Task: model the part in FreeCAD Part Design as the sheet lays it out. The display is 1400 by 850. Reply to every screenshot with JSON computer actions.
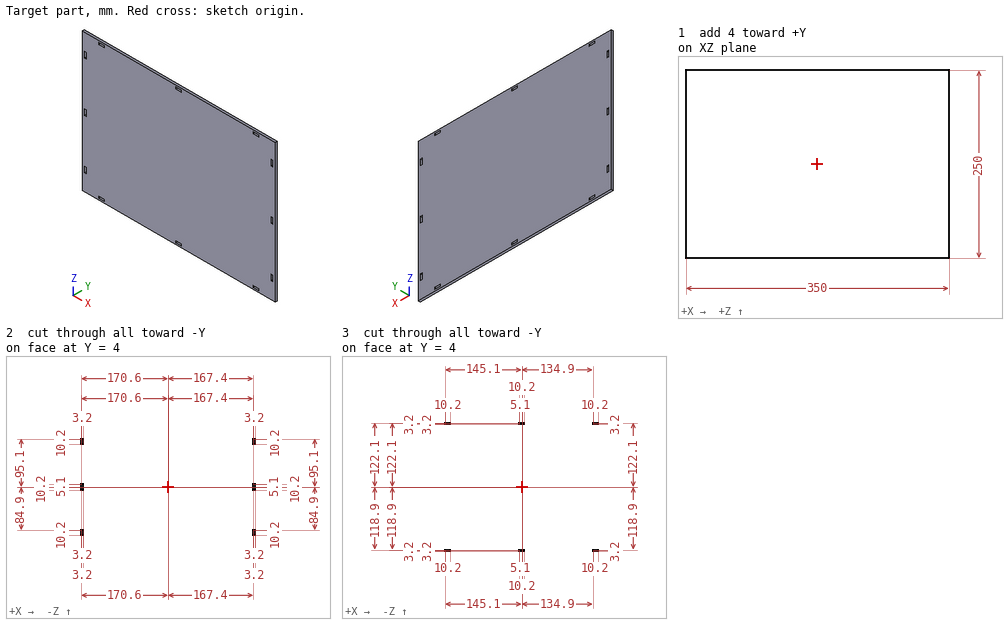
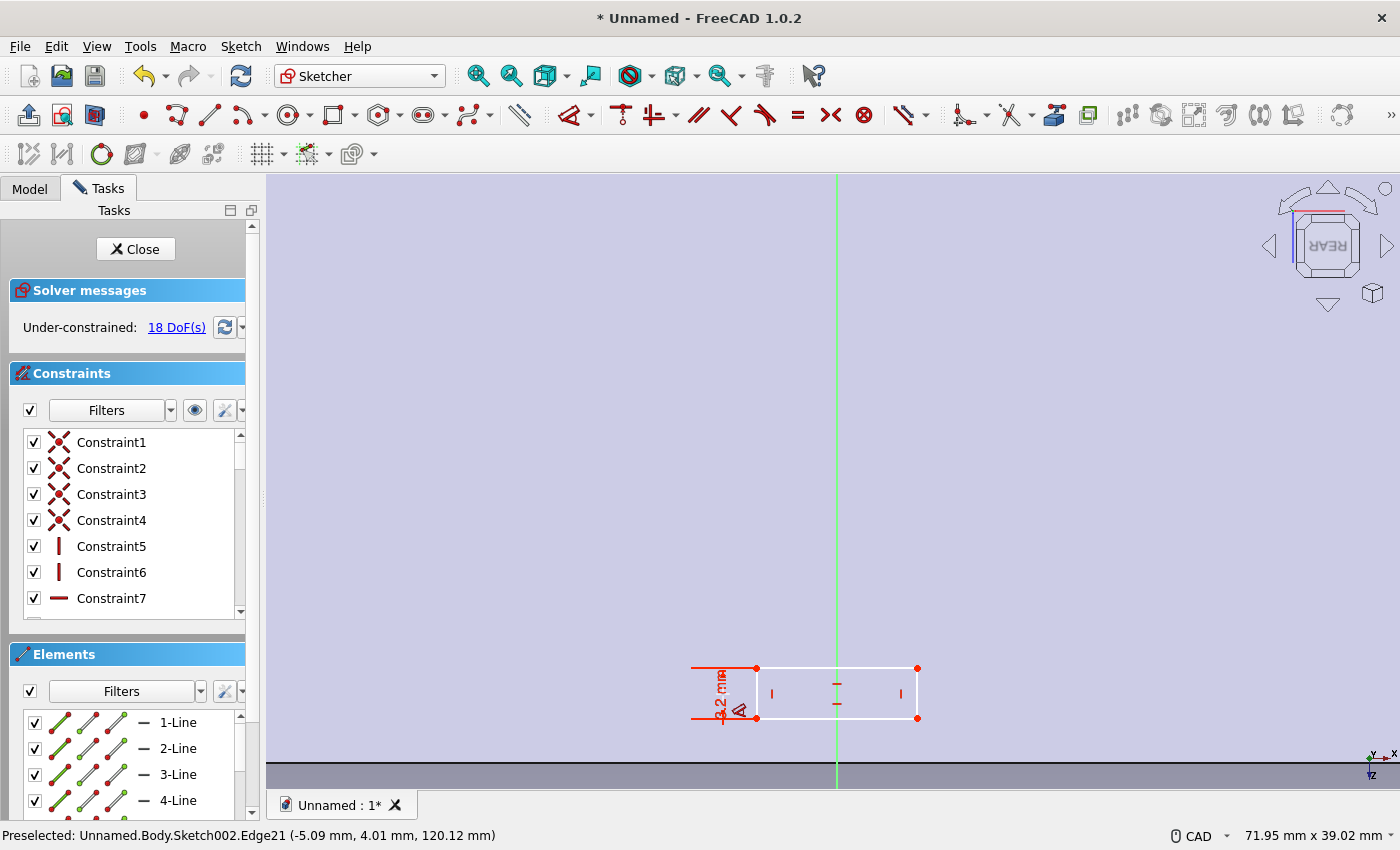
{"action": "scroll", "coordinate": [755, 692], "scroll_direction": "down", "scroll_amount": 11}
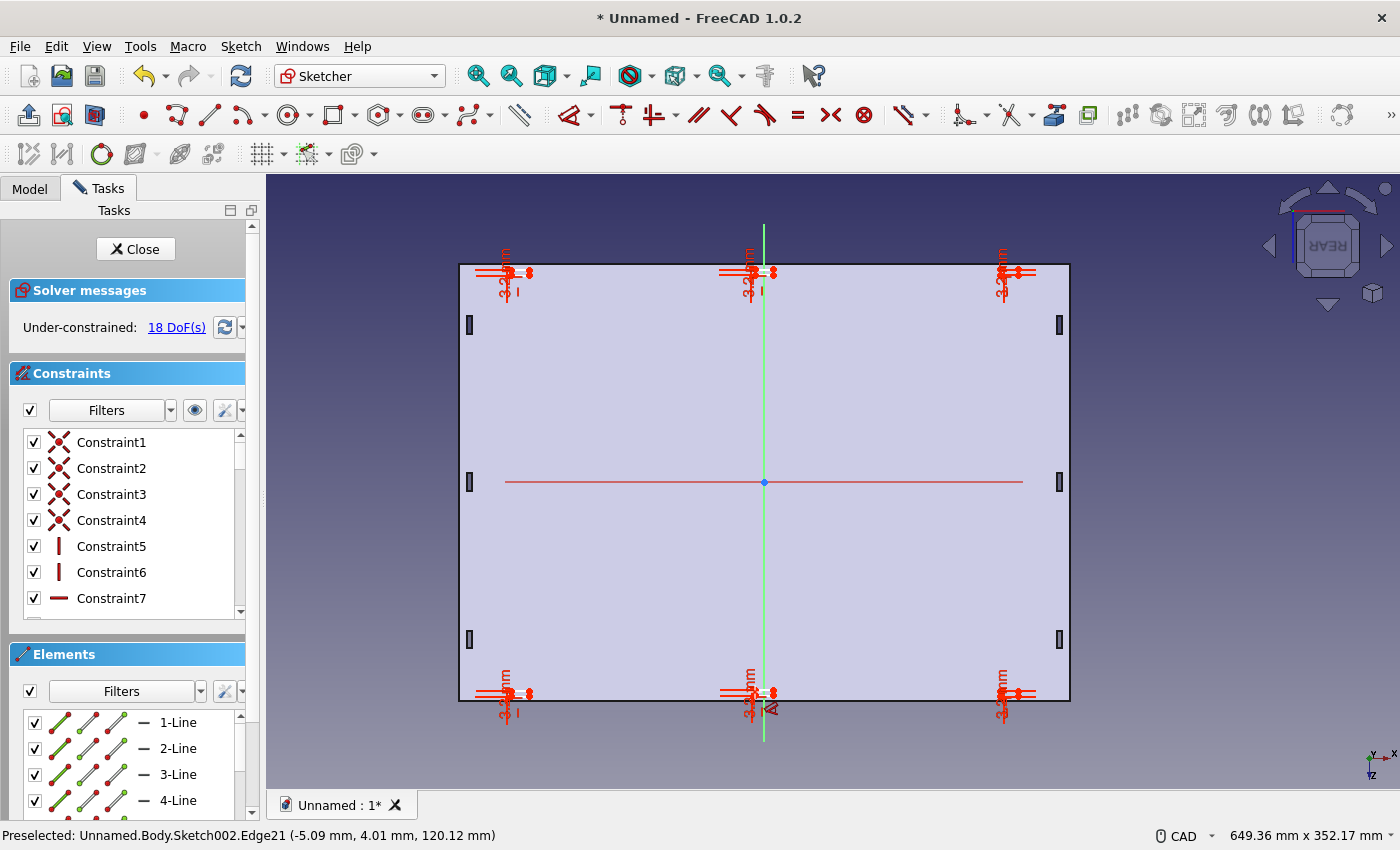
{"action": "scroll", "coordinate": [761, 275], "scroll_direction": "up", "scroll_amount": 7}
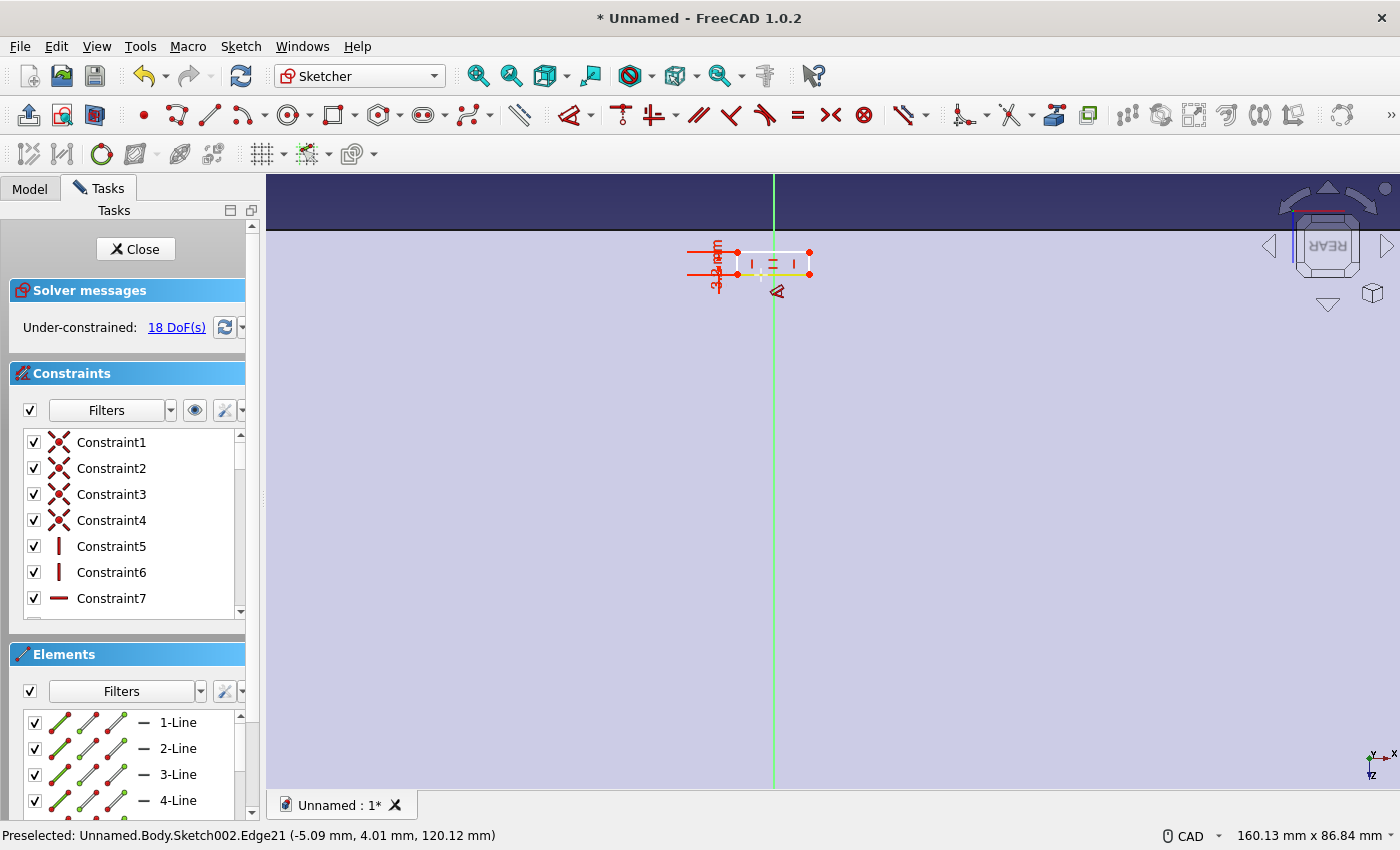
{"action": "left_click", "coordinate": [759, 275]}
{"action": "left_click", "coordinate": [757, 309]}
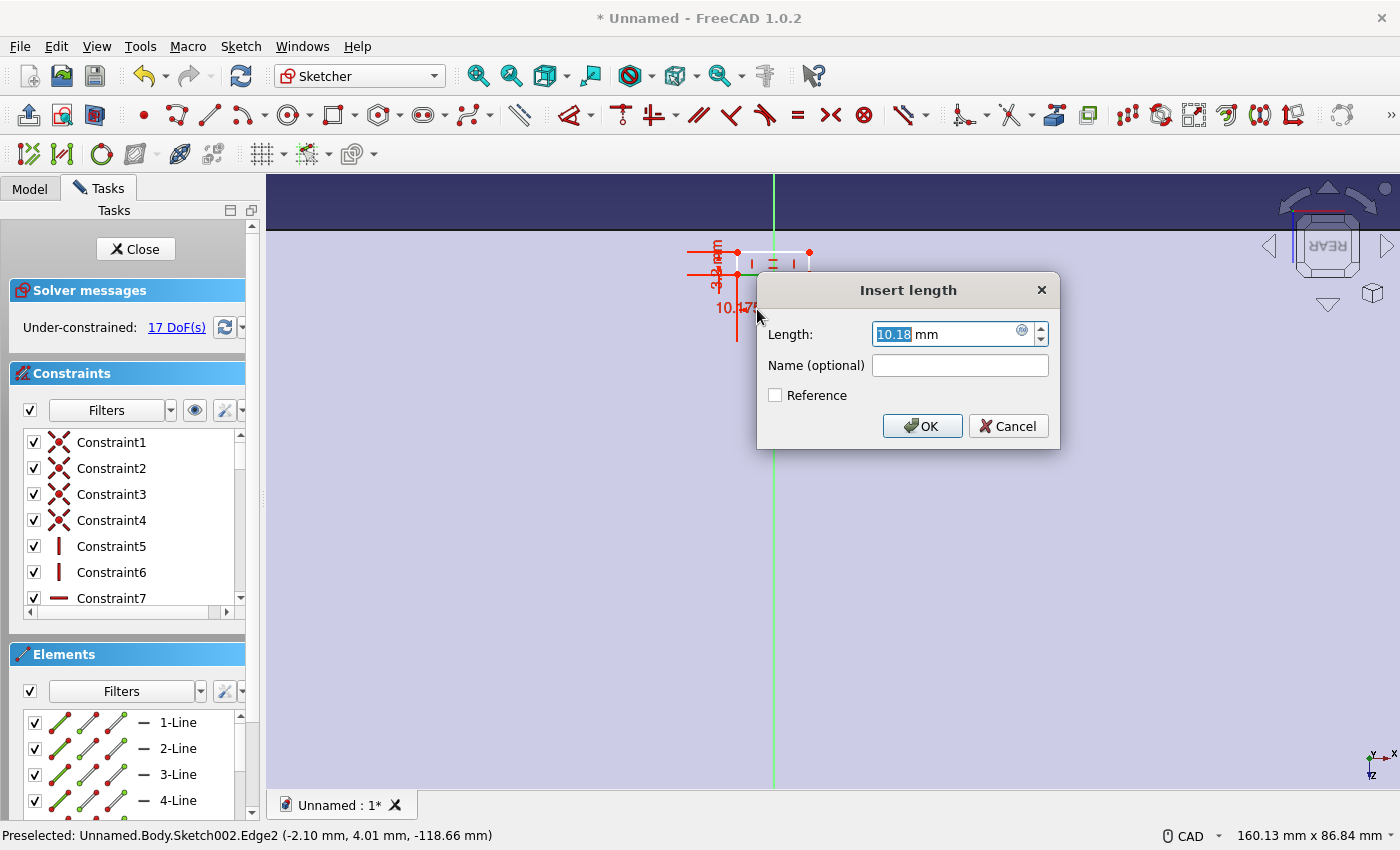
{"action": "type", "text": "10.2"}
{"action": "key", "text": "Return"}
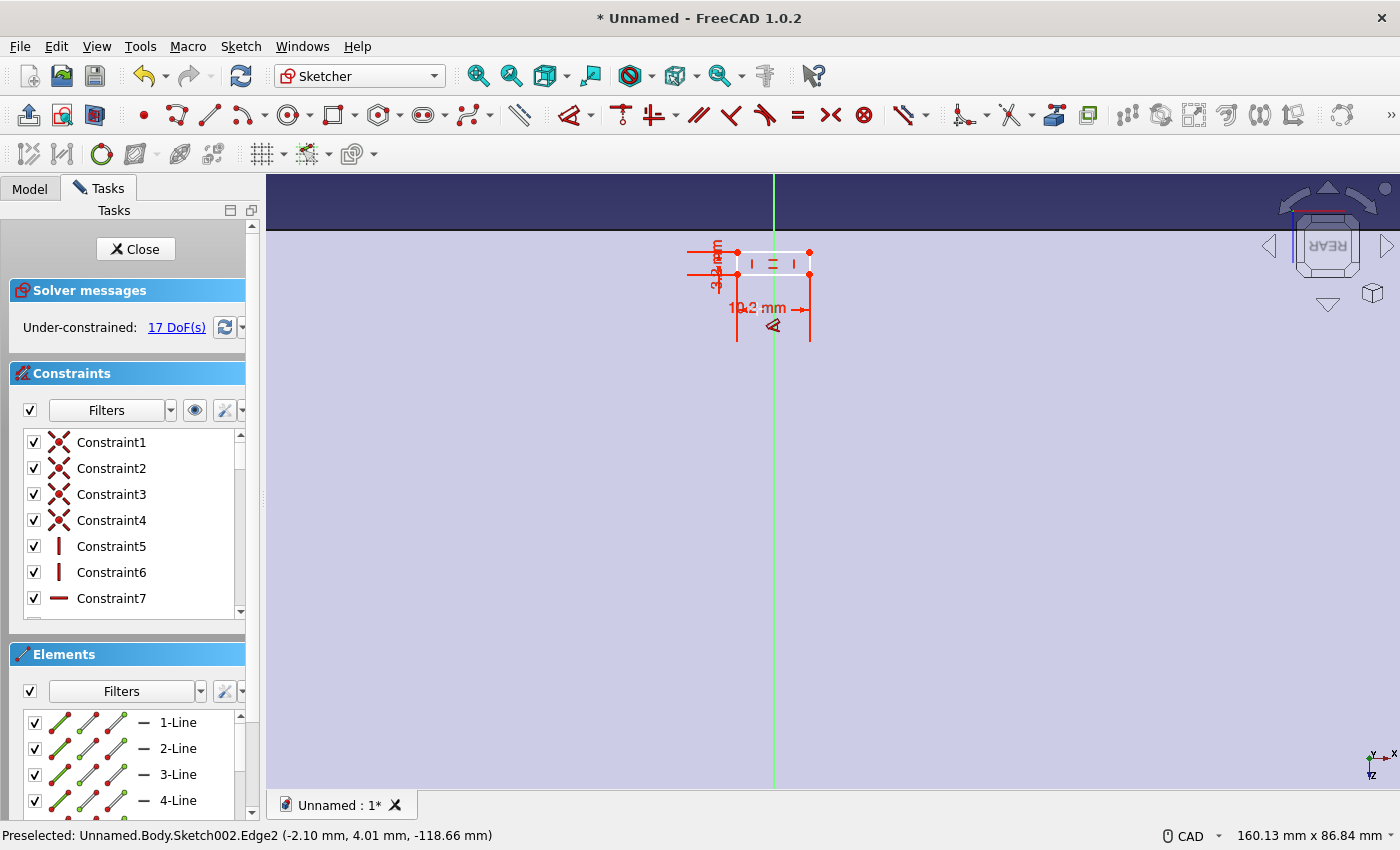
{"action": "scroll", "coordinate": [761, 274], "scroll_direction": "down", "scroll_amount": 7}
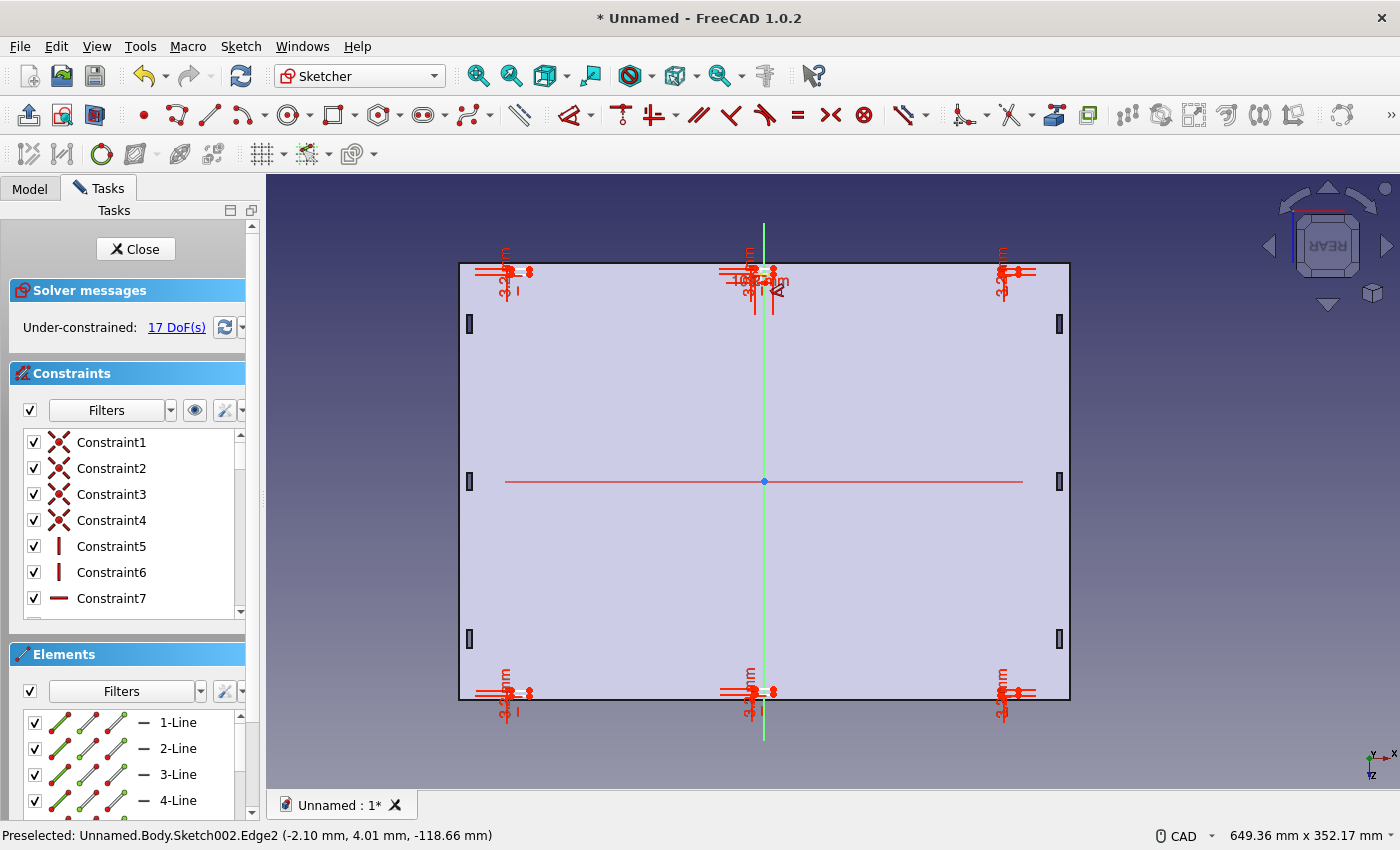
{"action": "scroll", "coordinate": [1006, 275], "scroll_direction": "up", "scroll_amount": 5}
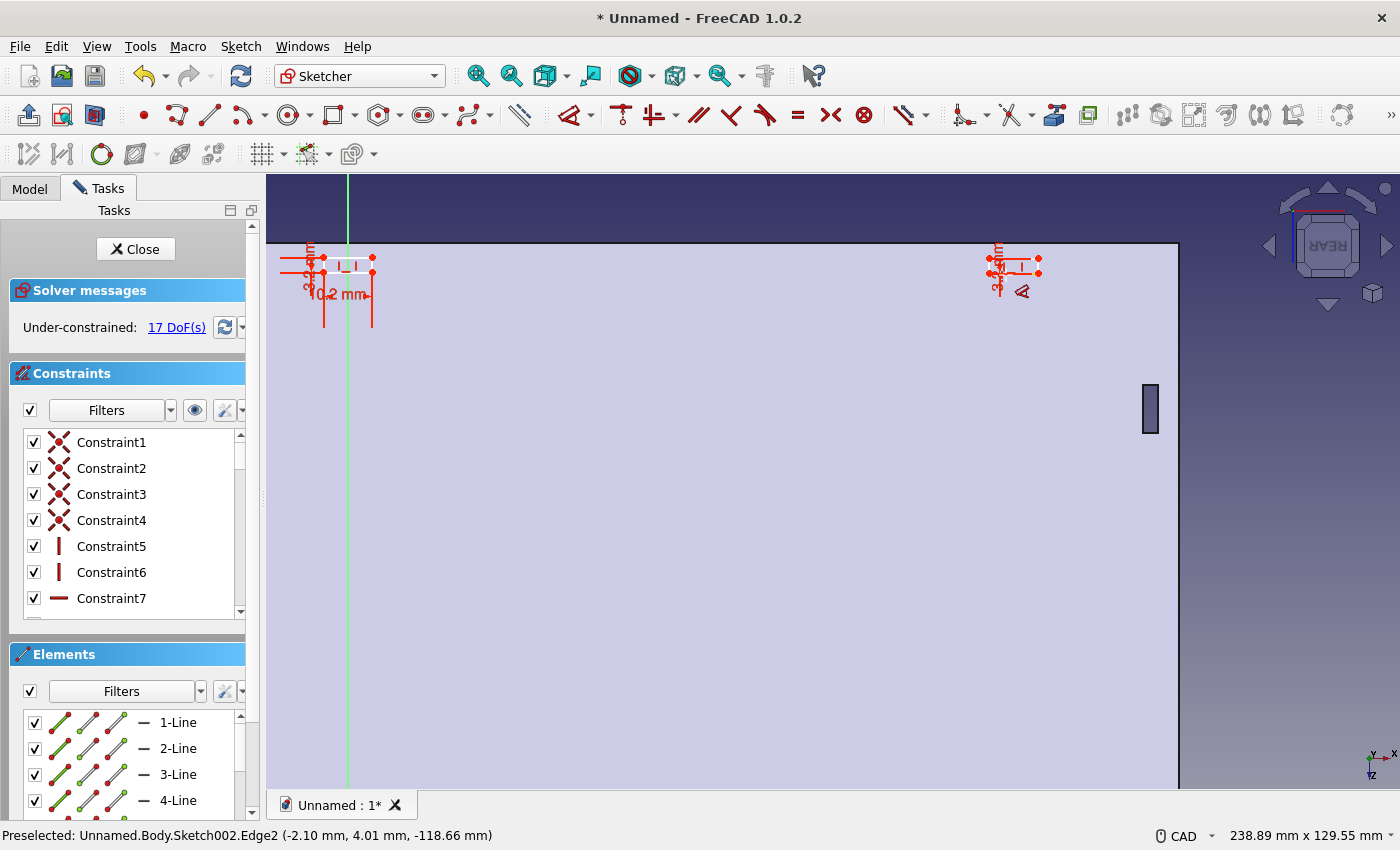
{"action": "left_click", "coordinate": [1004, 274]}
{"action": "left_click", "coordinate": [1014, 240]}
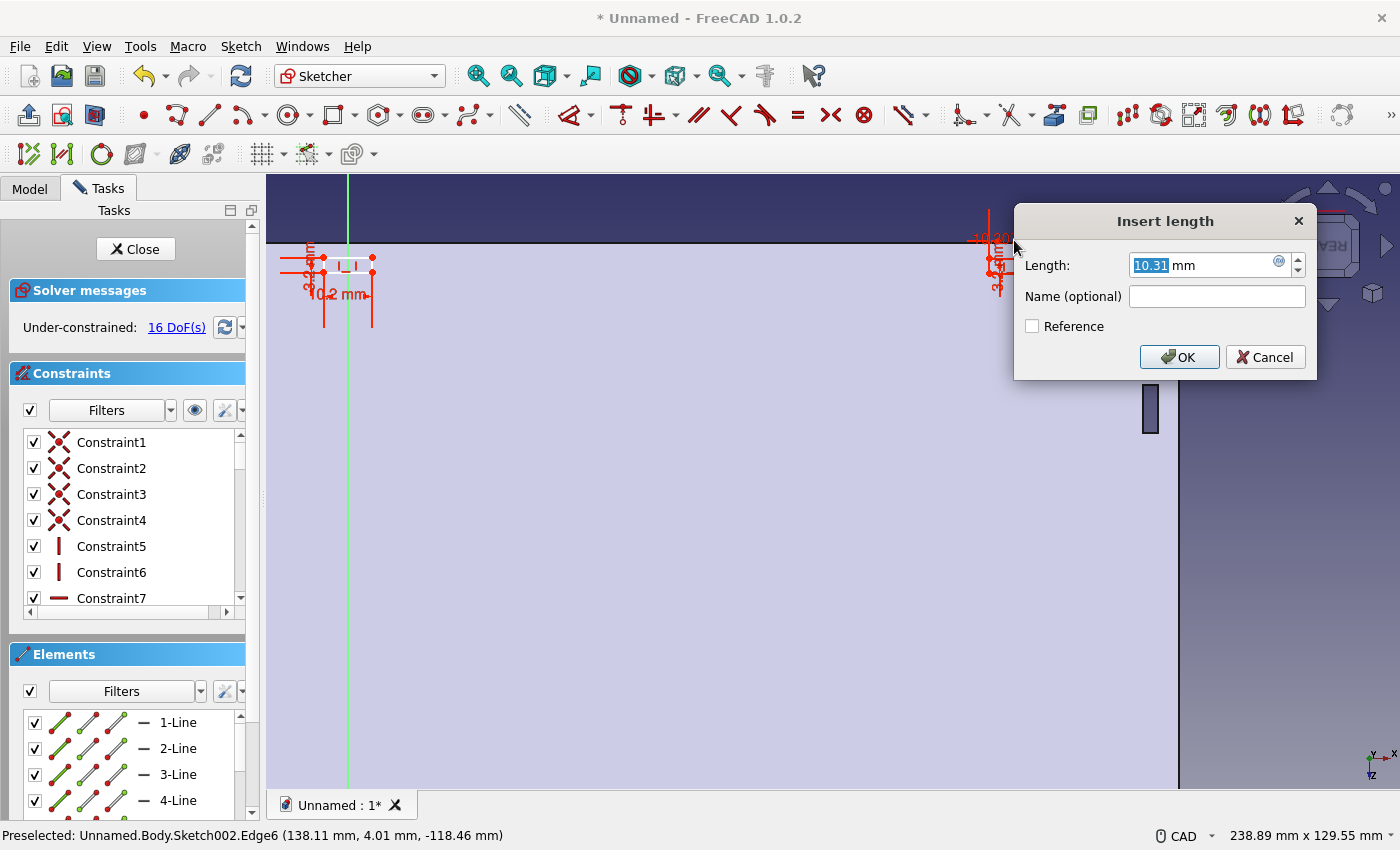
{"action": "type", "text": "10.2"}
{"action": "key", "text": "Return"}